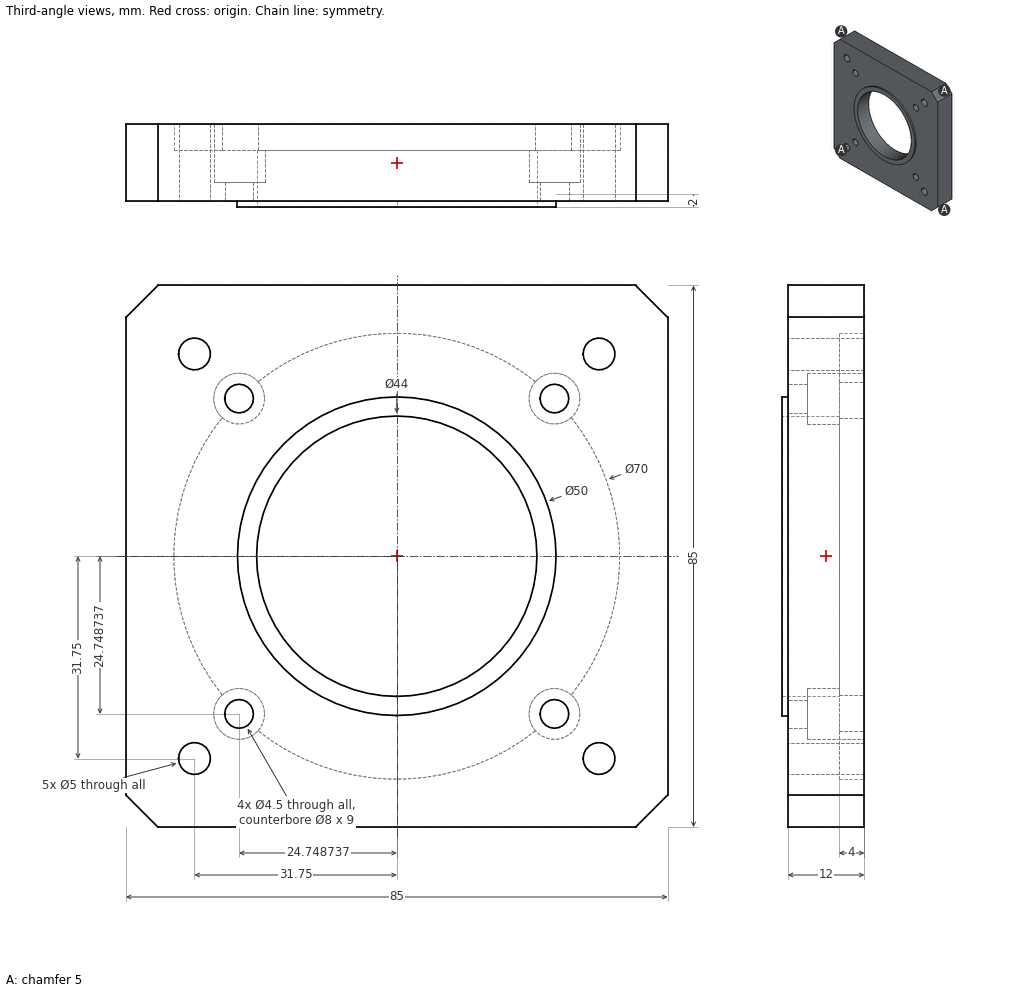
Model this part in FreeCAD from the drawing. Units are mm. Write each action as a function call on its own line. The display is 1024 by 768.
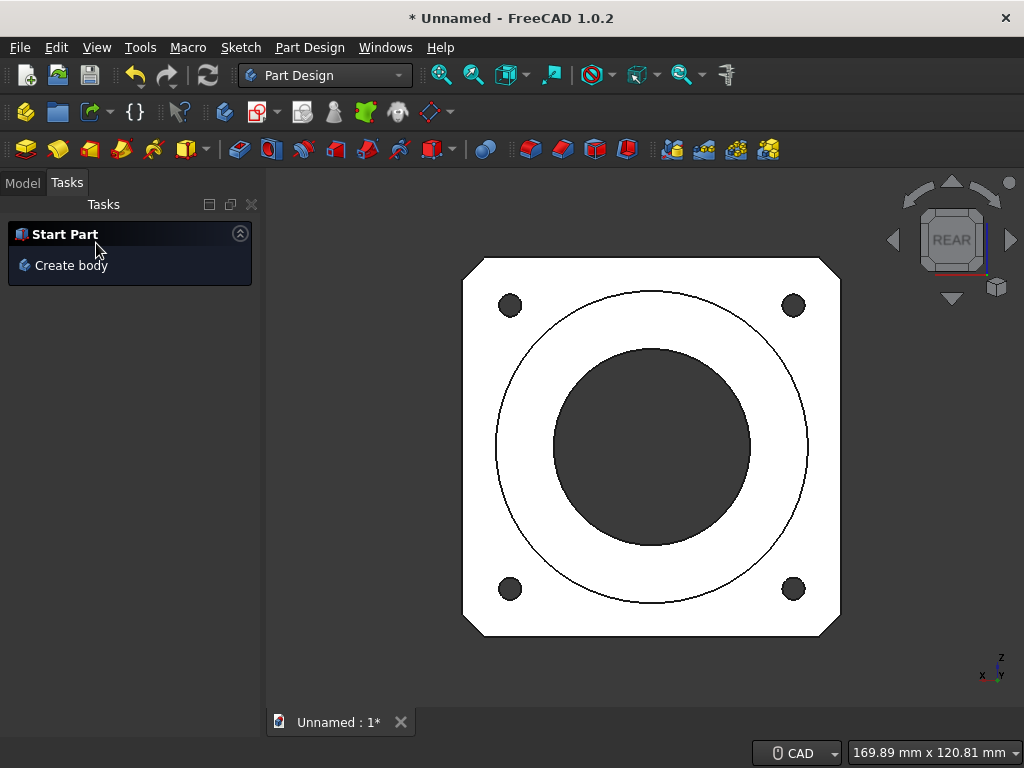
click(544, 609)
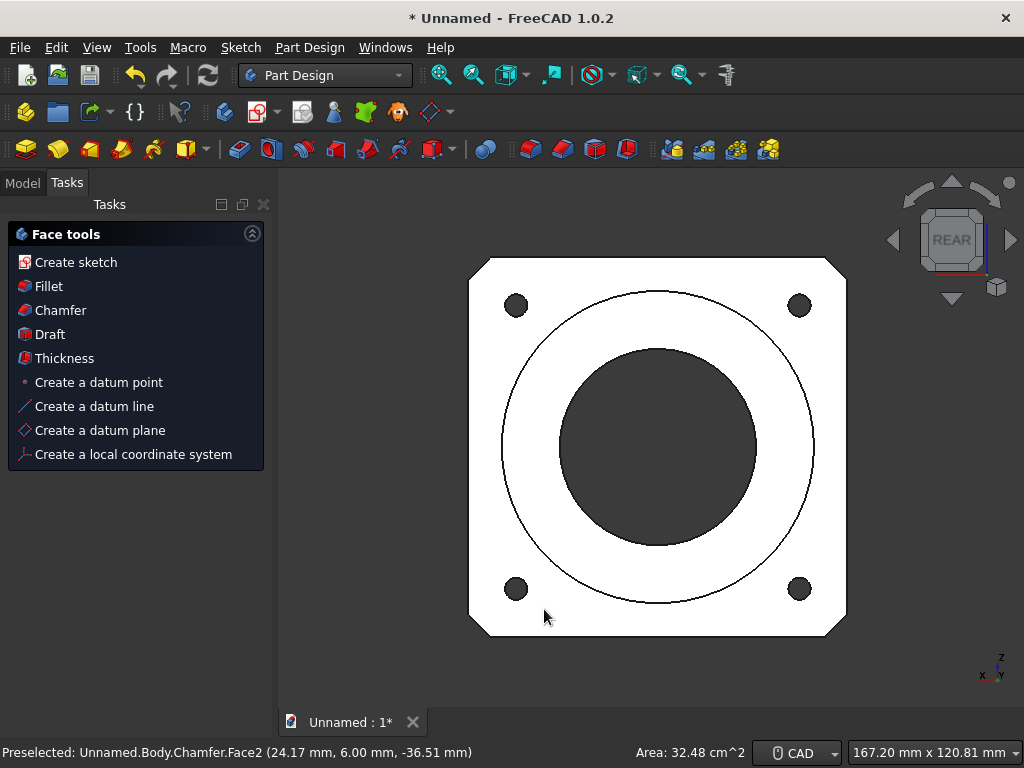
click(258, 112)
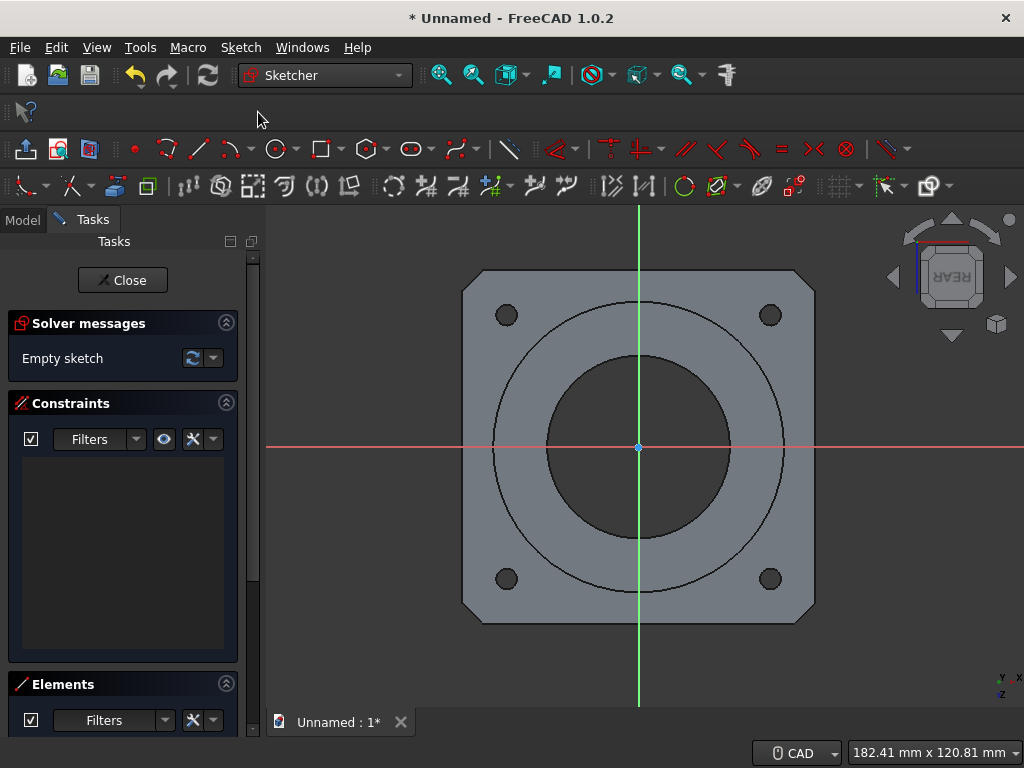
scroll(765, 429, up, 2)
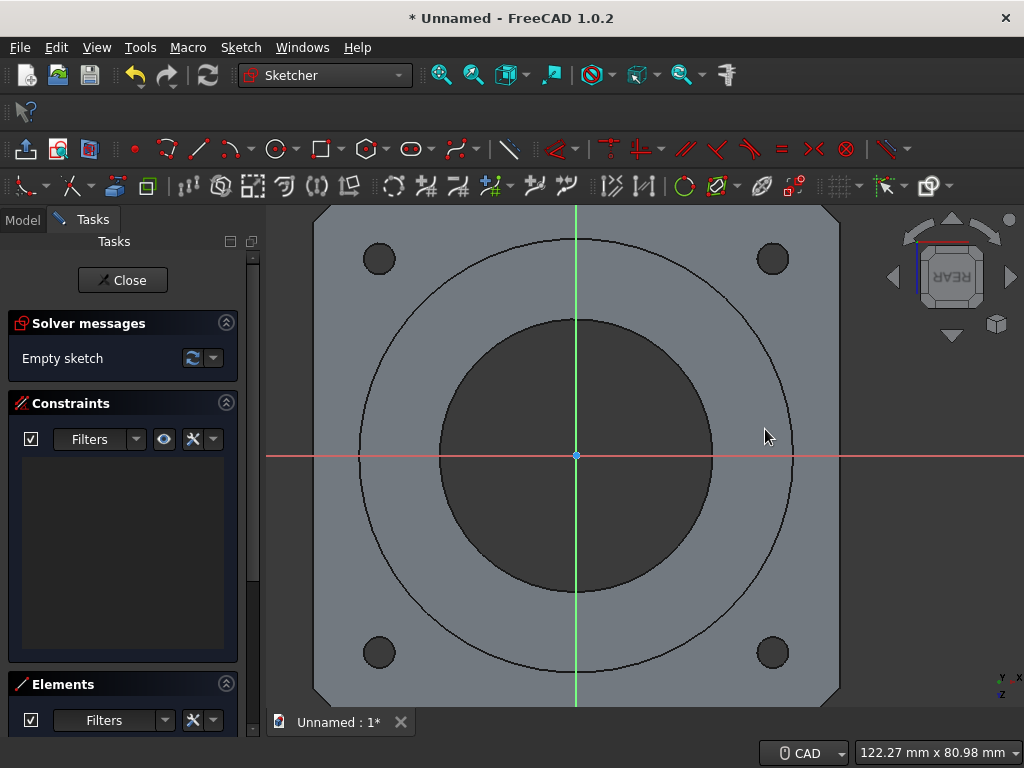
key(g)
key(c)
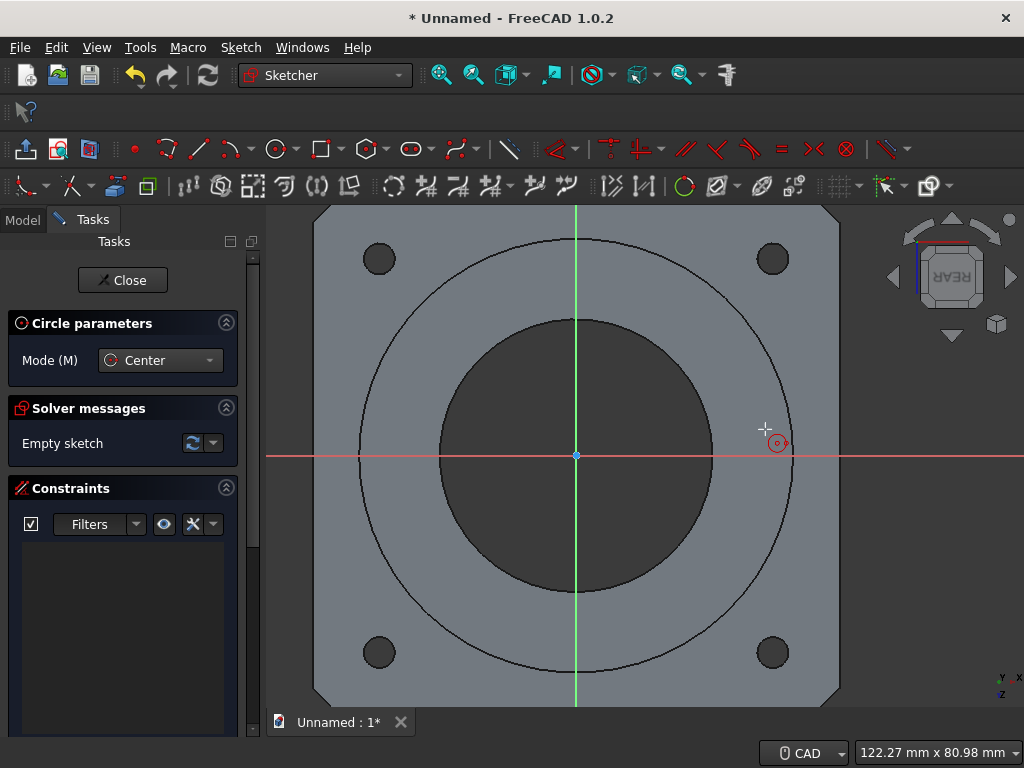
scroll(423, 302, up, 3)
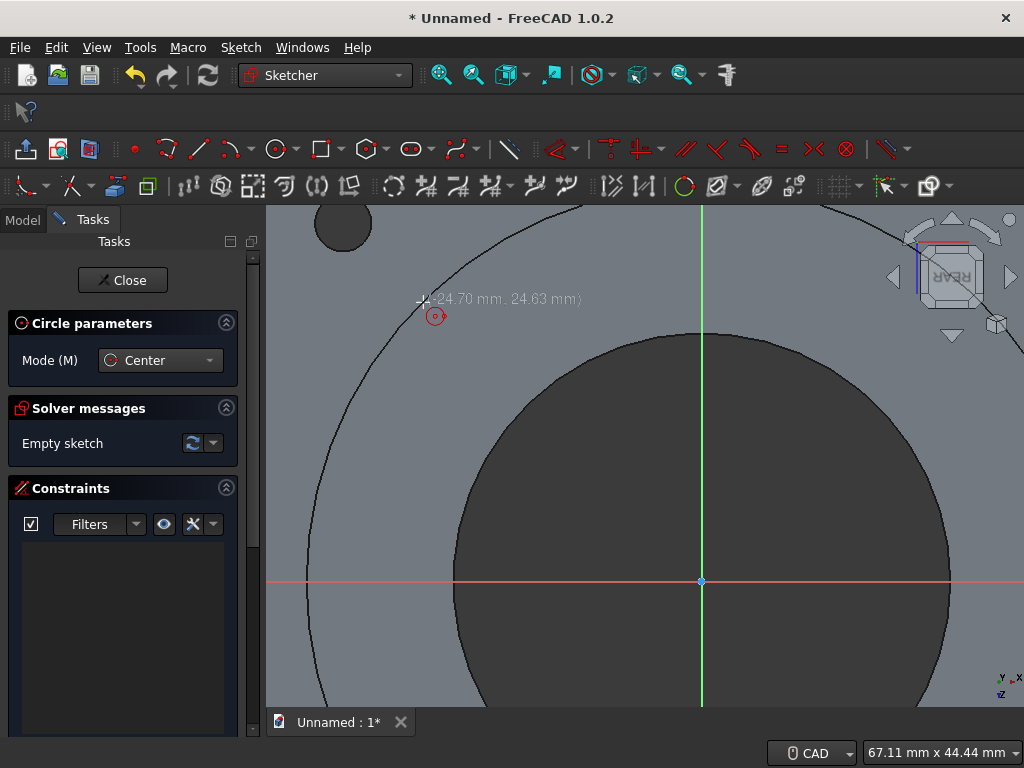
click(422, 302)
move(440, 284)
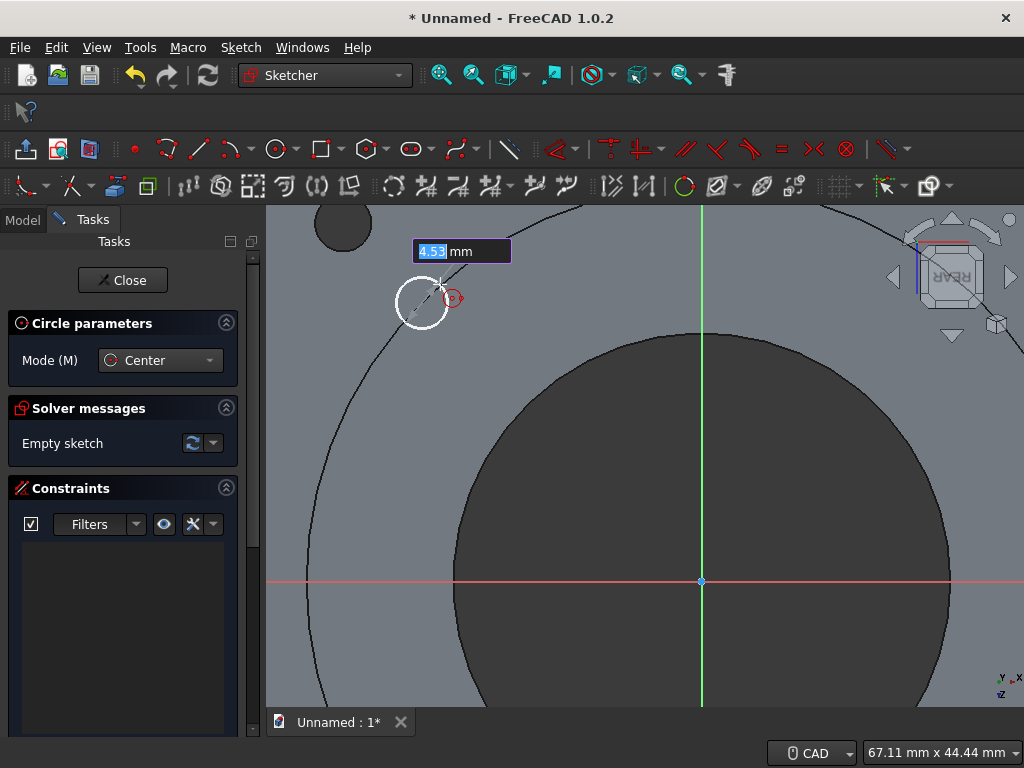
text(4.5)
key(Return)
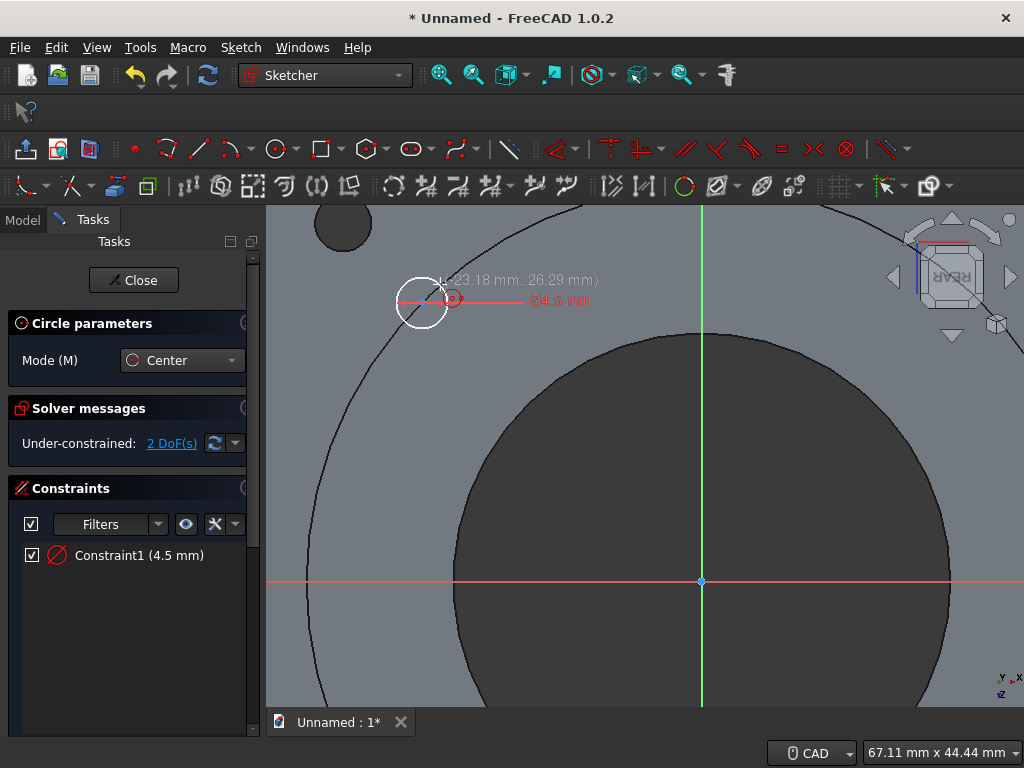
scroll(424, 303, down, 3)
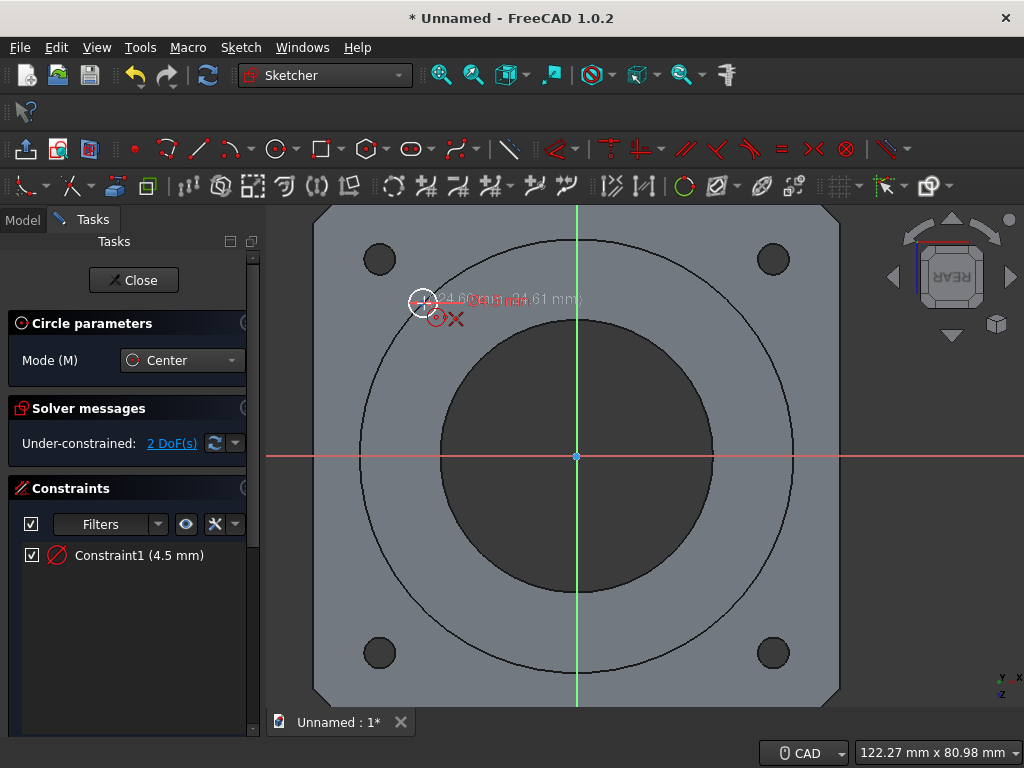
scroll(730, 303, up, 3)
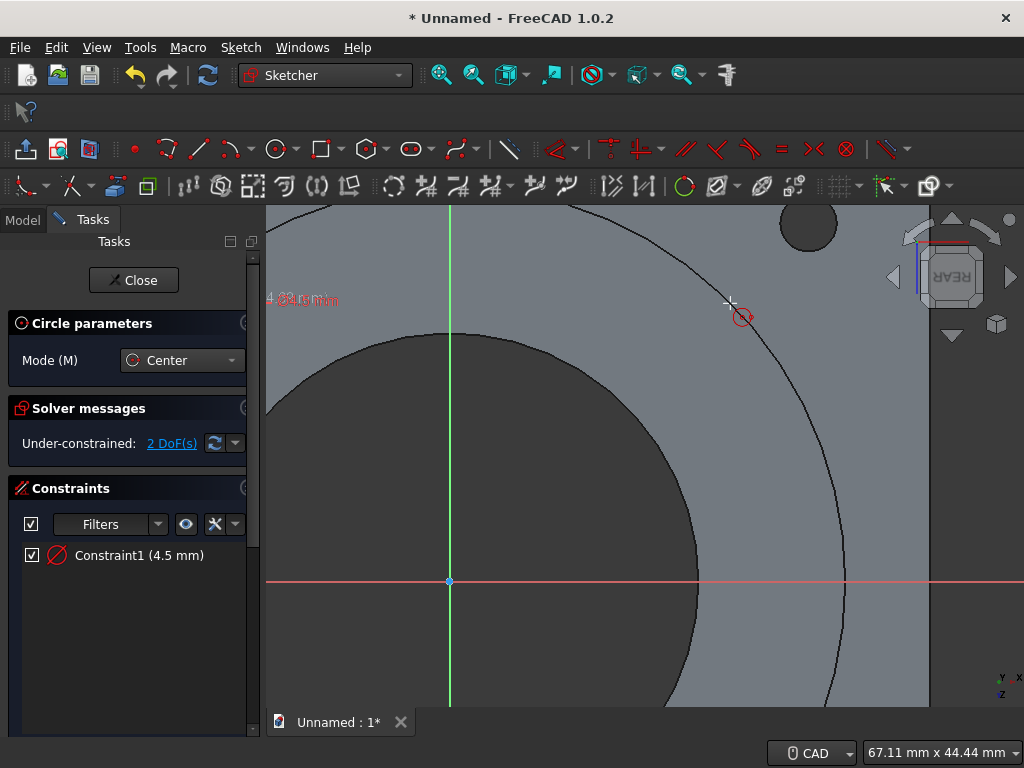
click(730, 302)
move(747, 284)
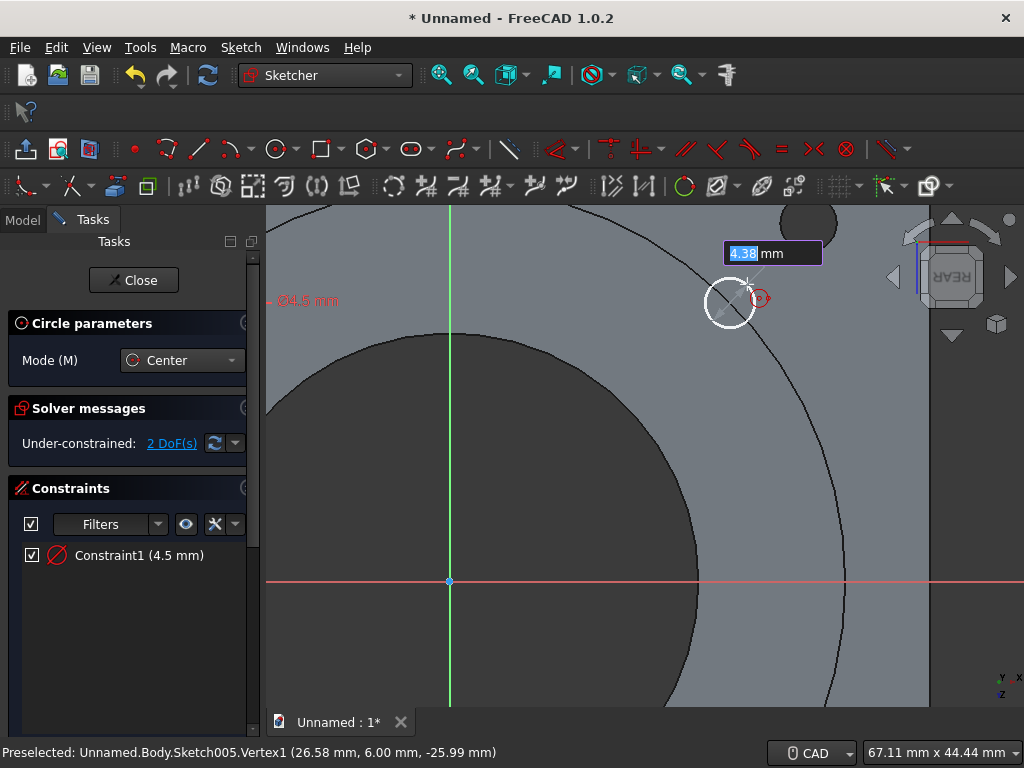
text(4.5)
key(Return)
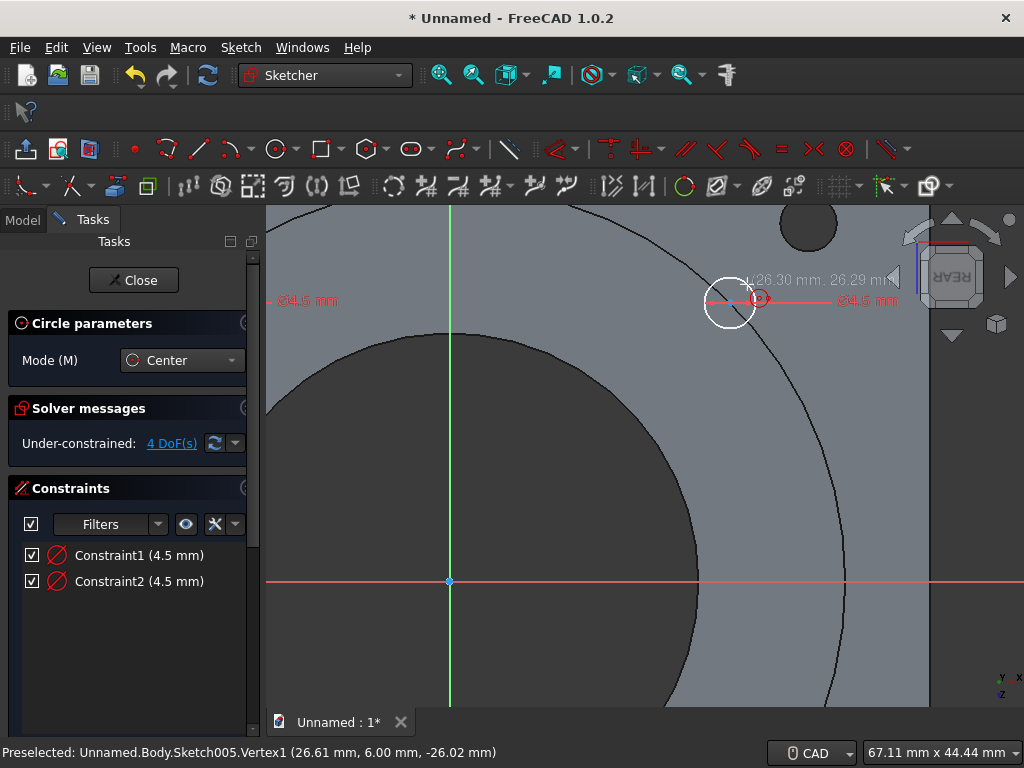
scroll(730, 303, down, 3)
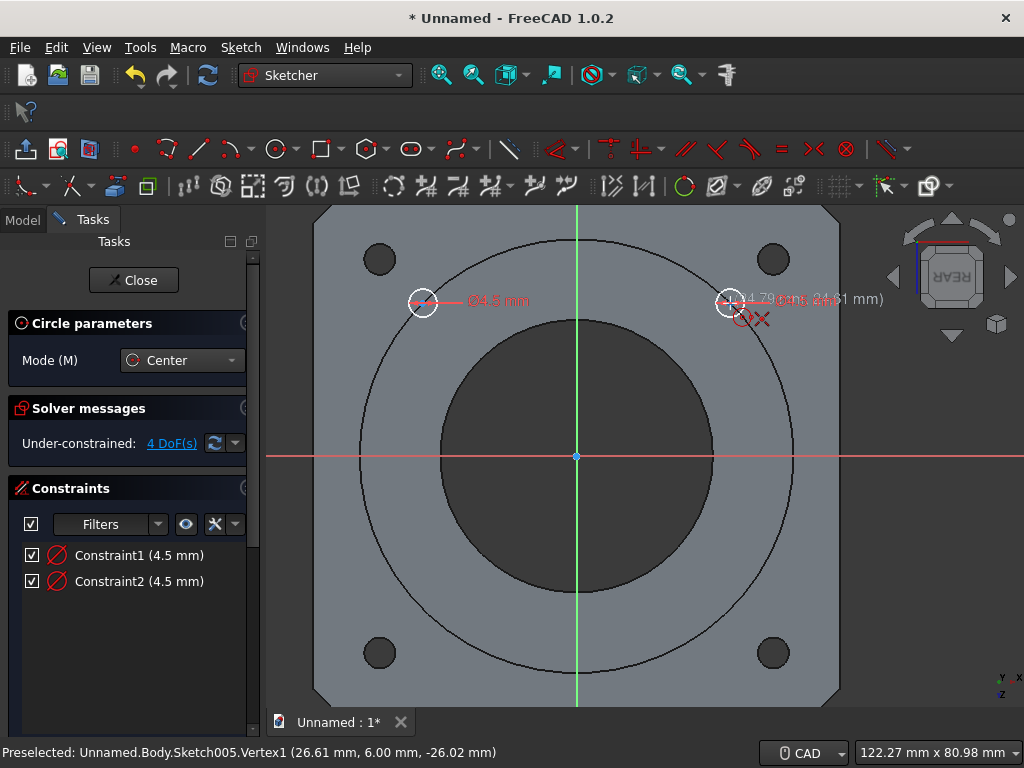
scroll(730, 610, up, 3)